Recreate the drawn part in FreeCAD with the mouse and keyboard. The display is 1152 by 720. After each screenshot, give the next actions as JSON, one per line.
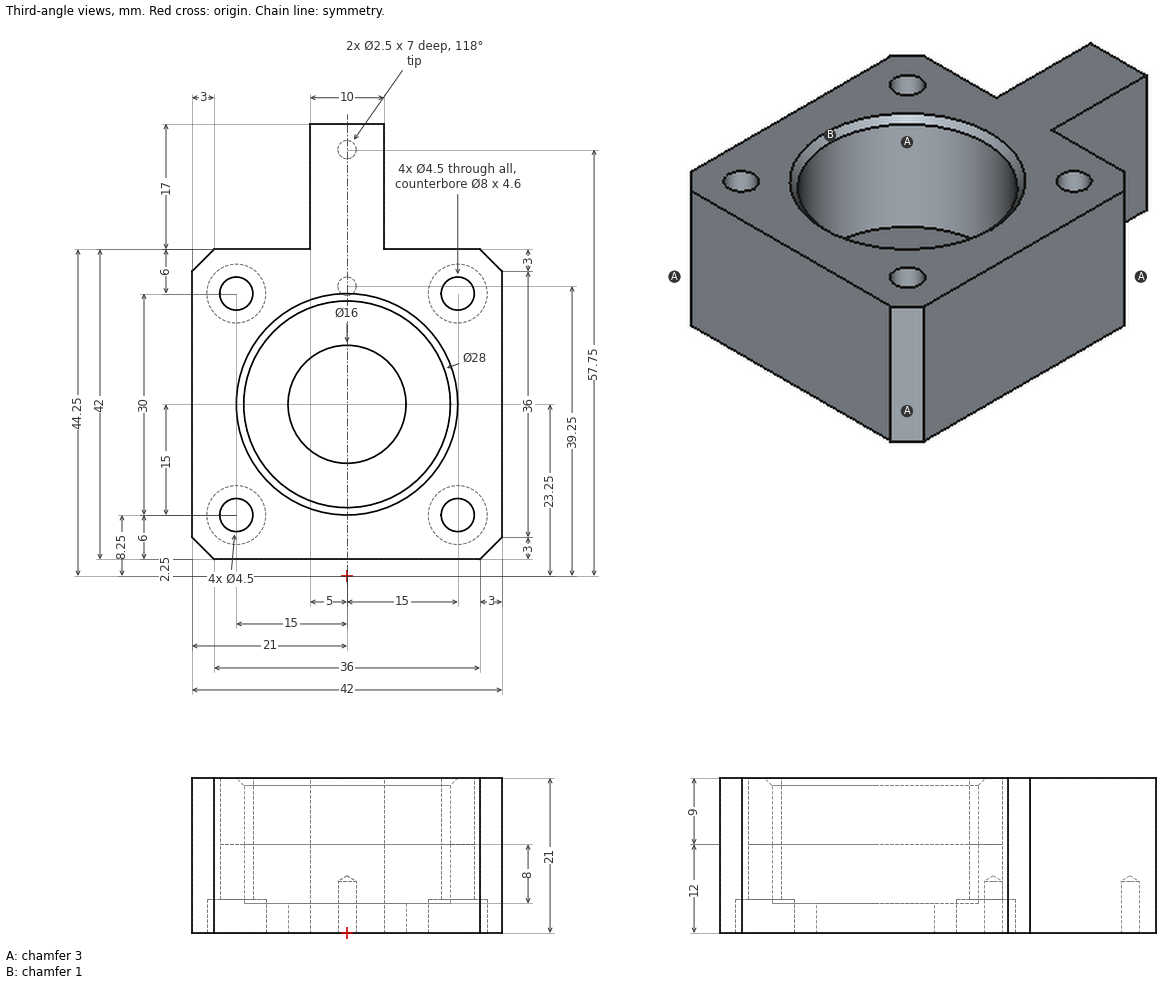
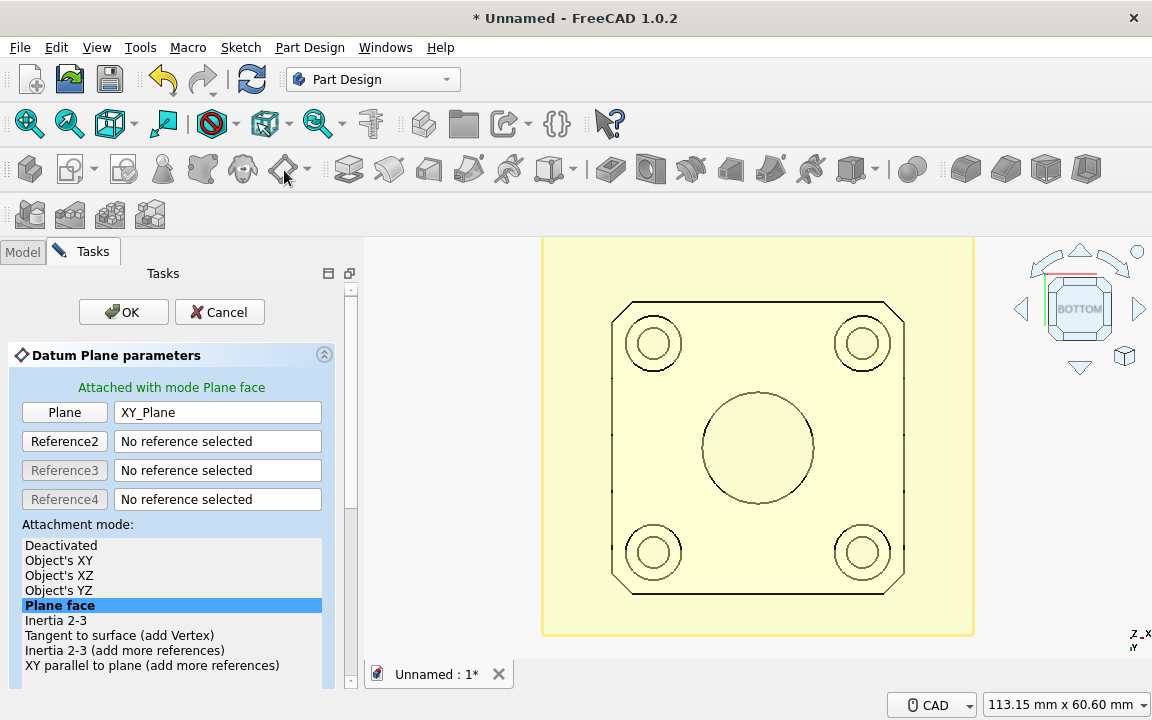
{"action": "scroll", "coordinate": [351, 486], "scroll_direction": "down", "scroll_amount": 4}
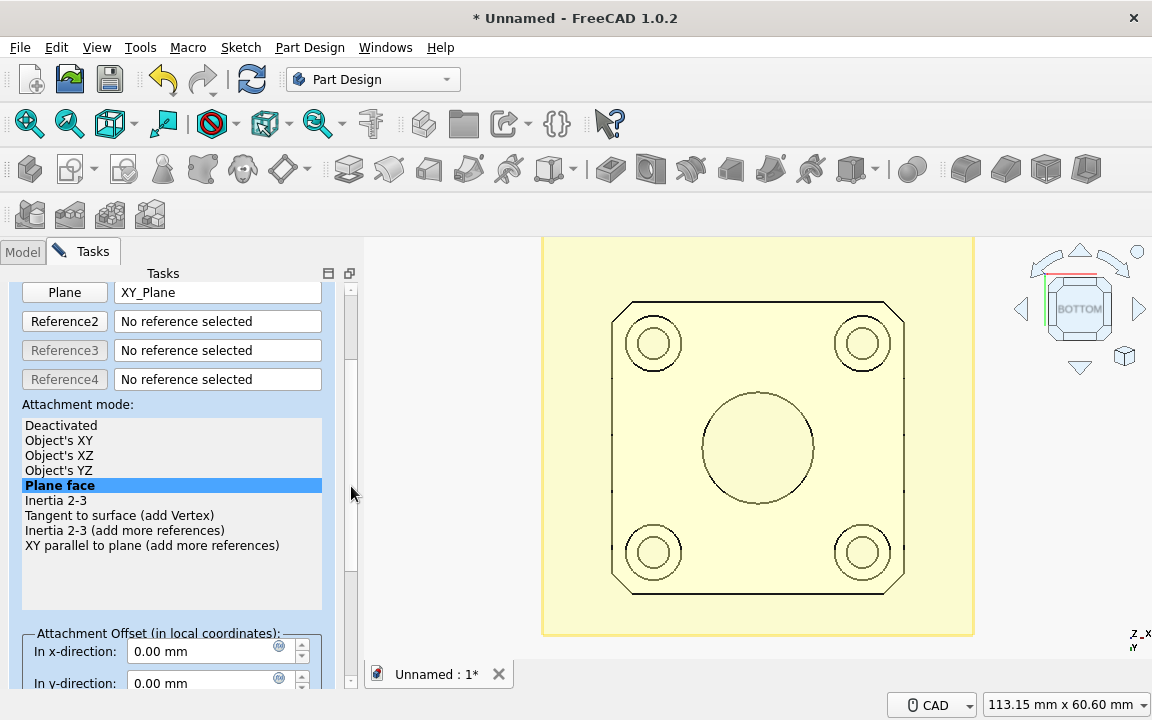
{"action": "triple_click", "coordinate": [210, 595]}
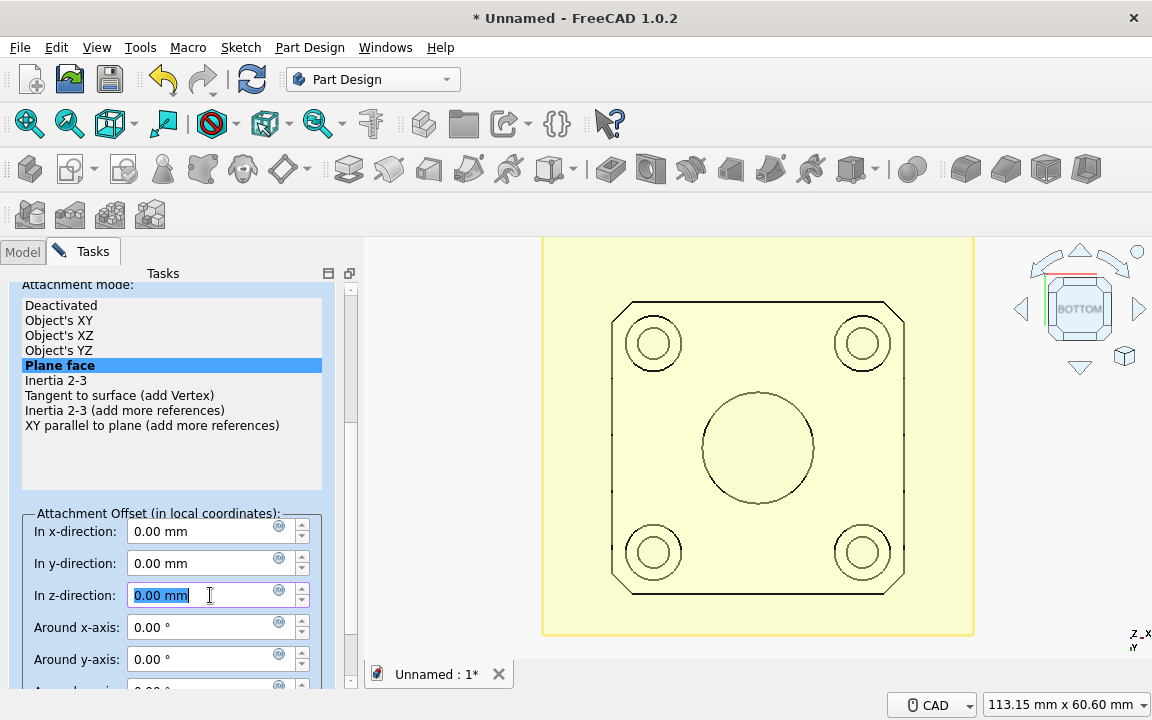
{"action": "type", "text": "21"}
{"action": "key", "text": "Tab"}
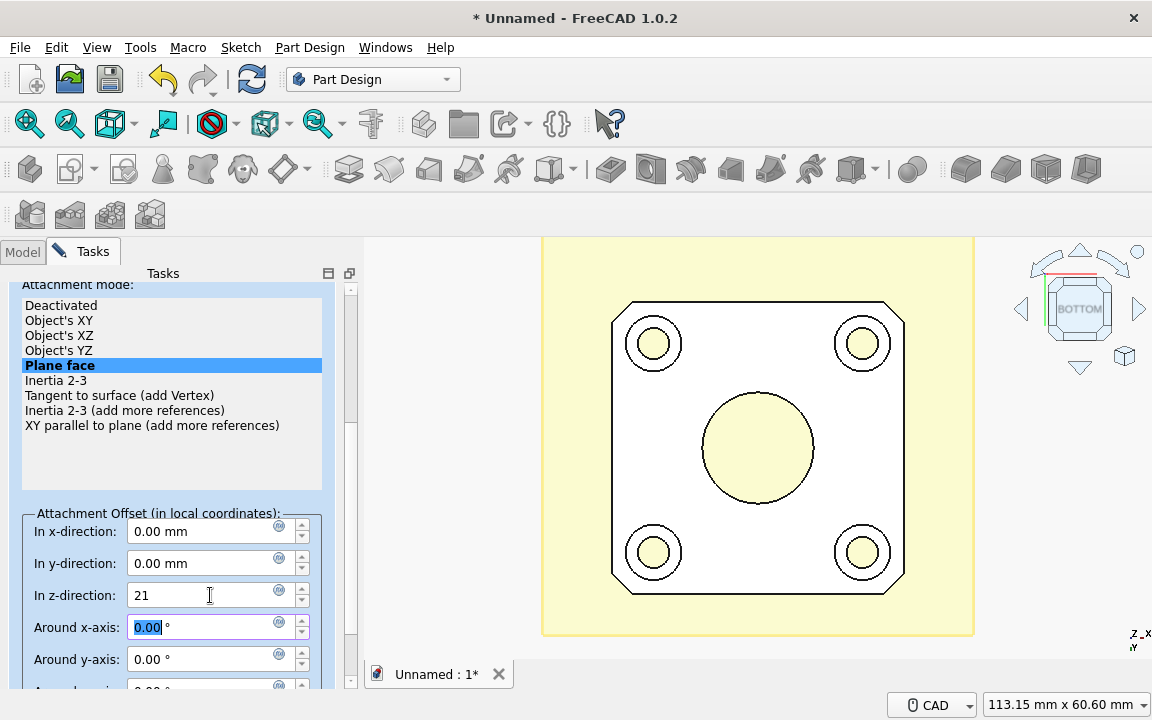
{"action": "scroll", "coordinate": [351, 486], "scroll_direction": "up", "scroll_amount": 5}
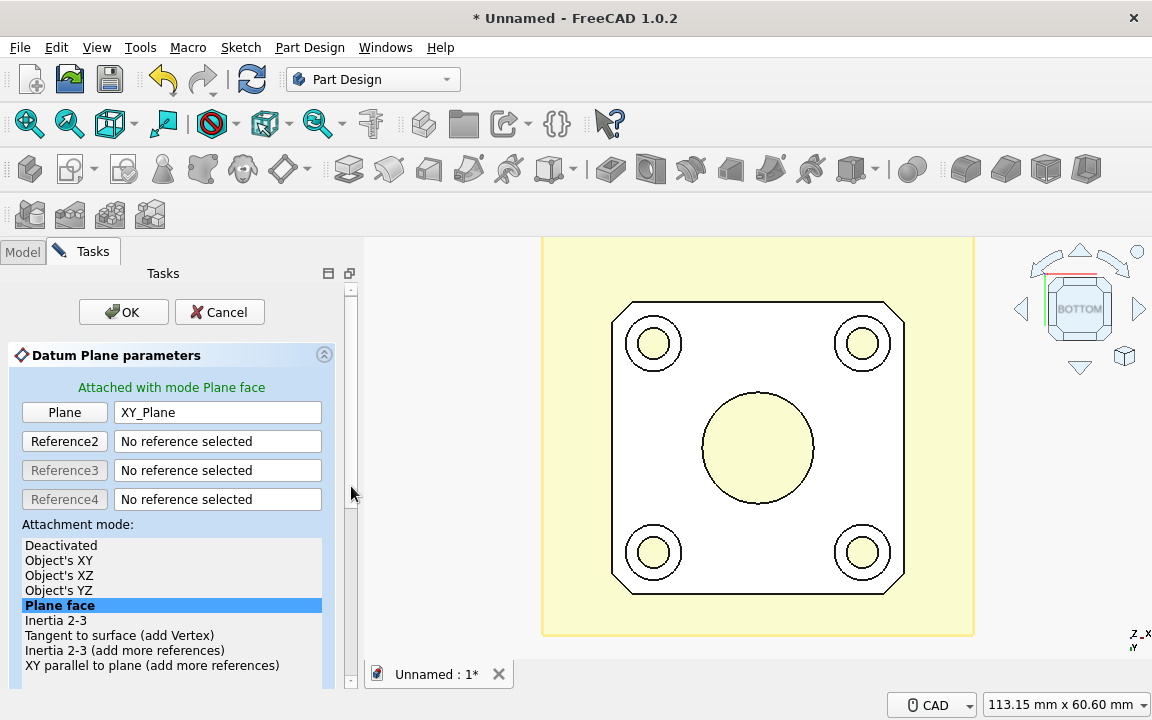
{"action": "left_click", "coordinate": [124, 312]}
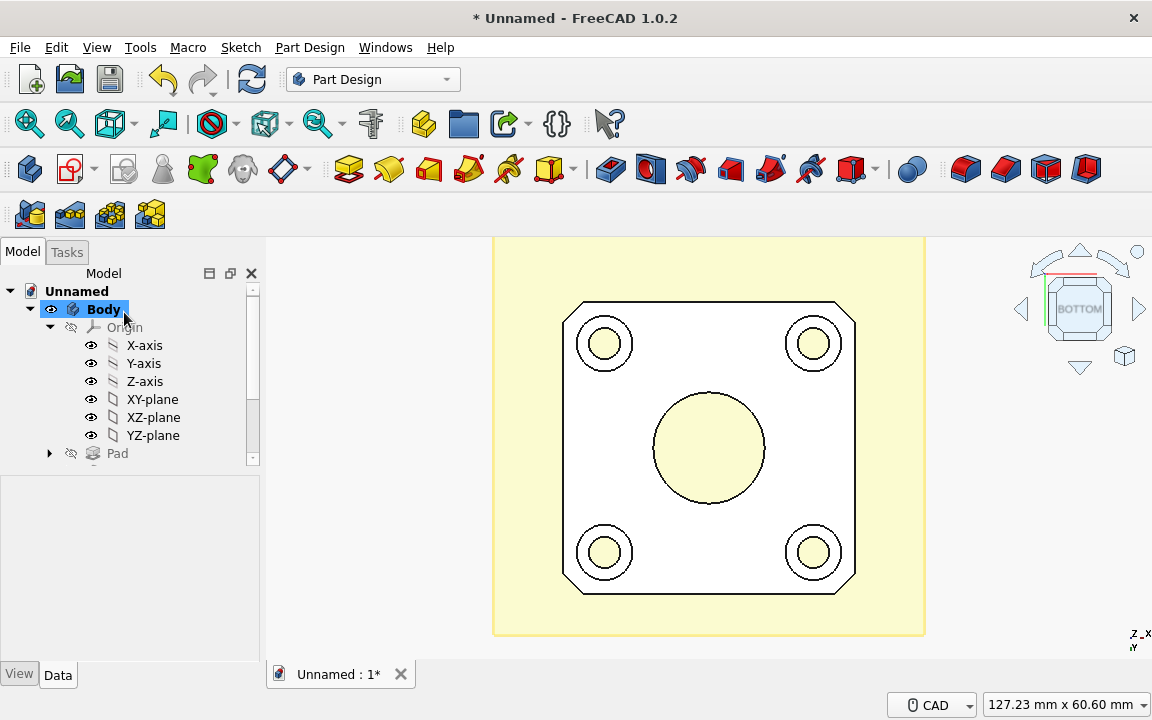
{"action": "scroll", "coordinate": [100, 377], "scroll_direction": "down", "scroll_amount": 3}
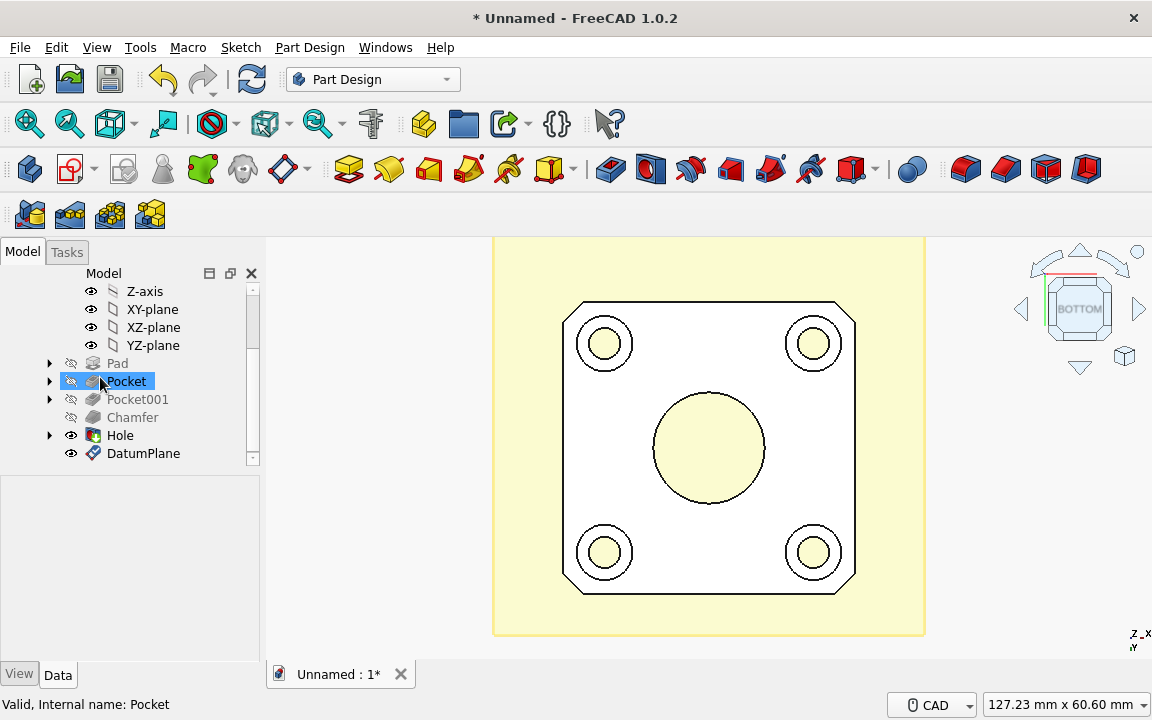
{"action": "left_click", "coordinate": [116, 453]}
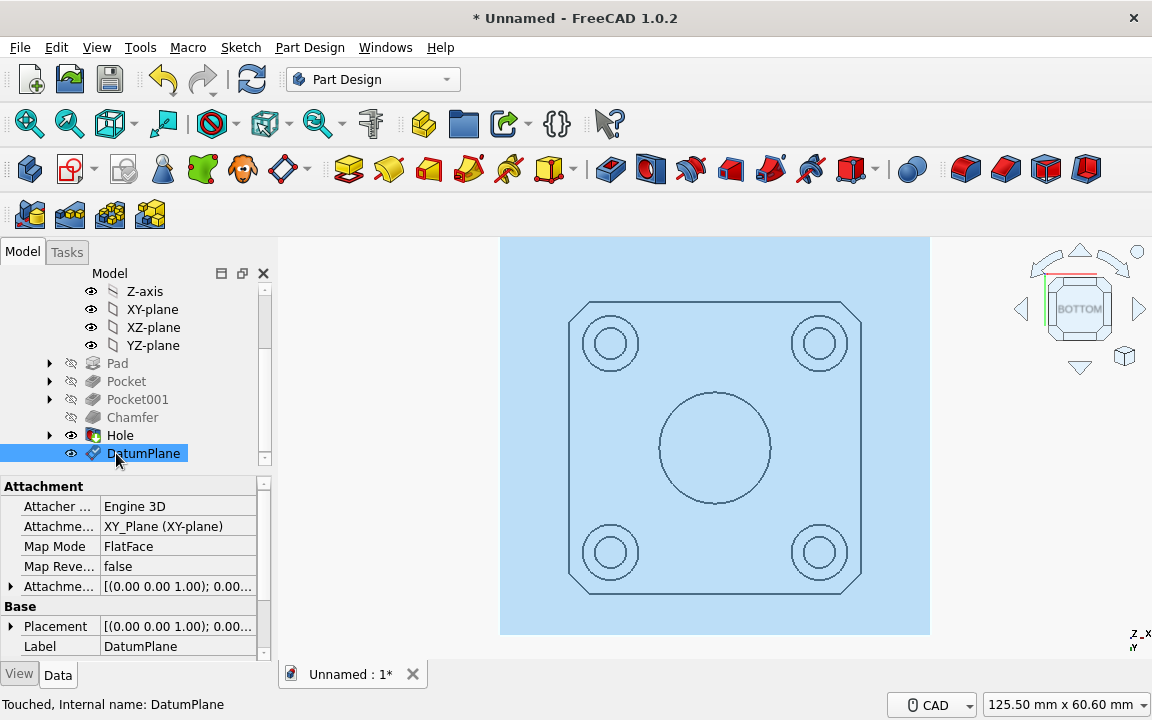
{"action": "left_click", "coordinate": [70, 170]}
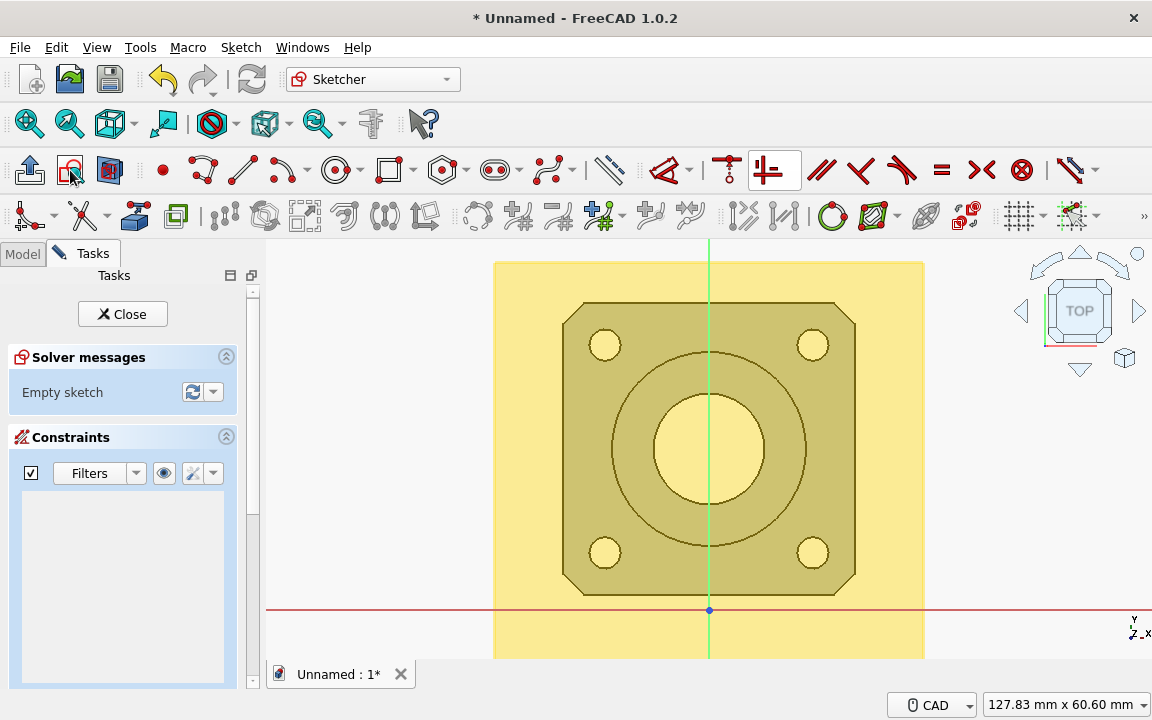
{"action": "scroll", "coordinate": [331, 414], "scroll_direction": "down", "scroll_amount": 1}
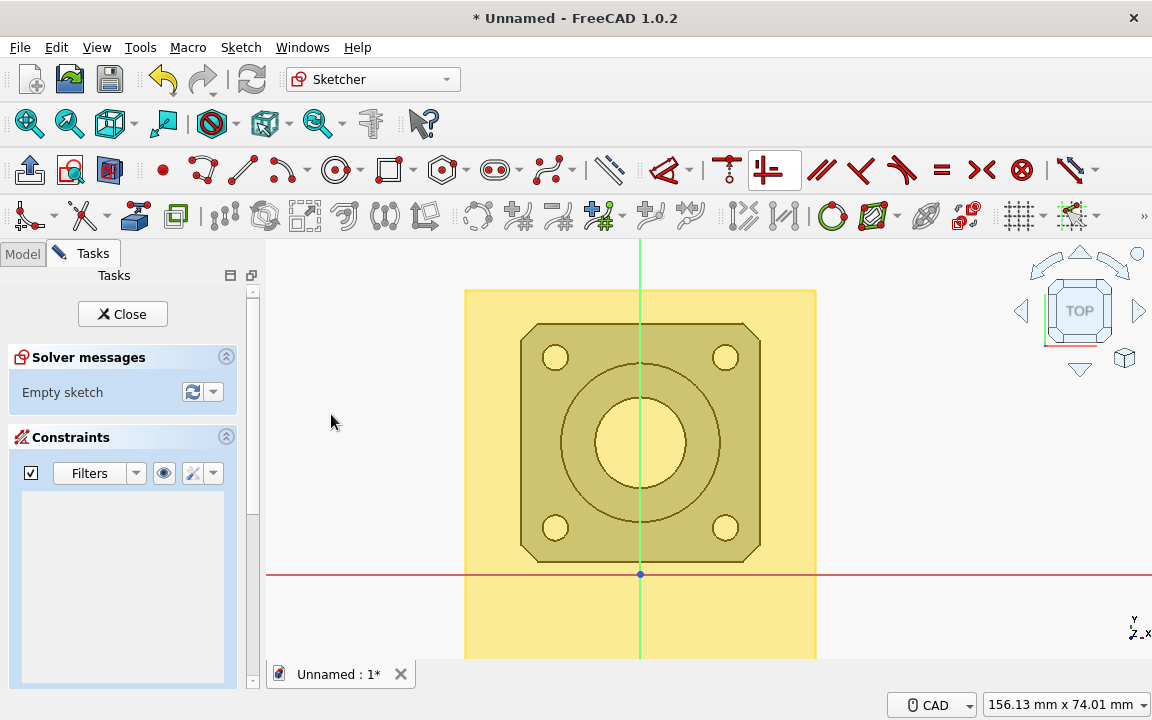
{"action": "left_click", "coordinate": [204, 170]}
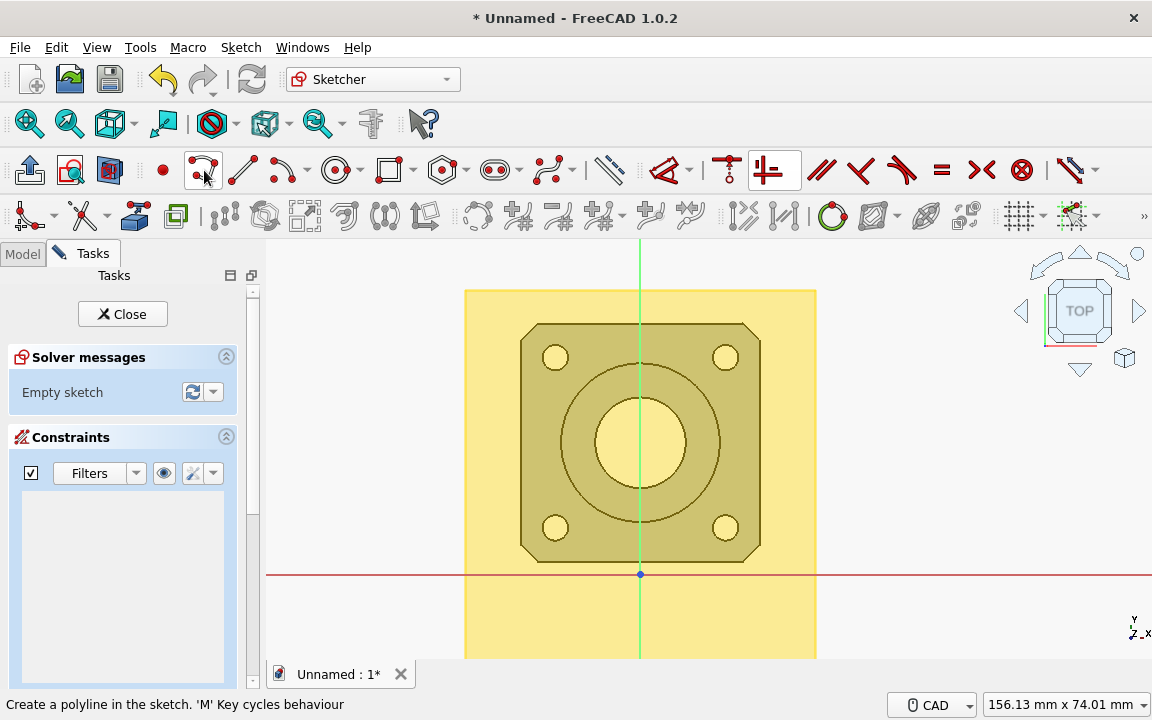
{"action": "scroll", "coordinate": [538, 562], "scroll_direction": "up", "scroll_amount": 2}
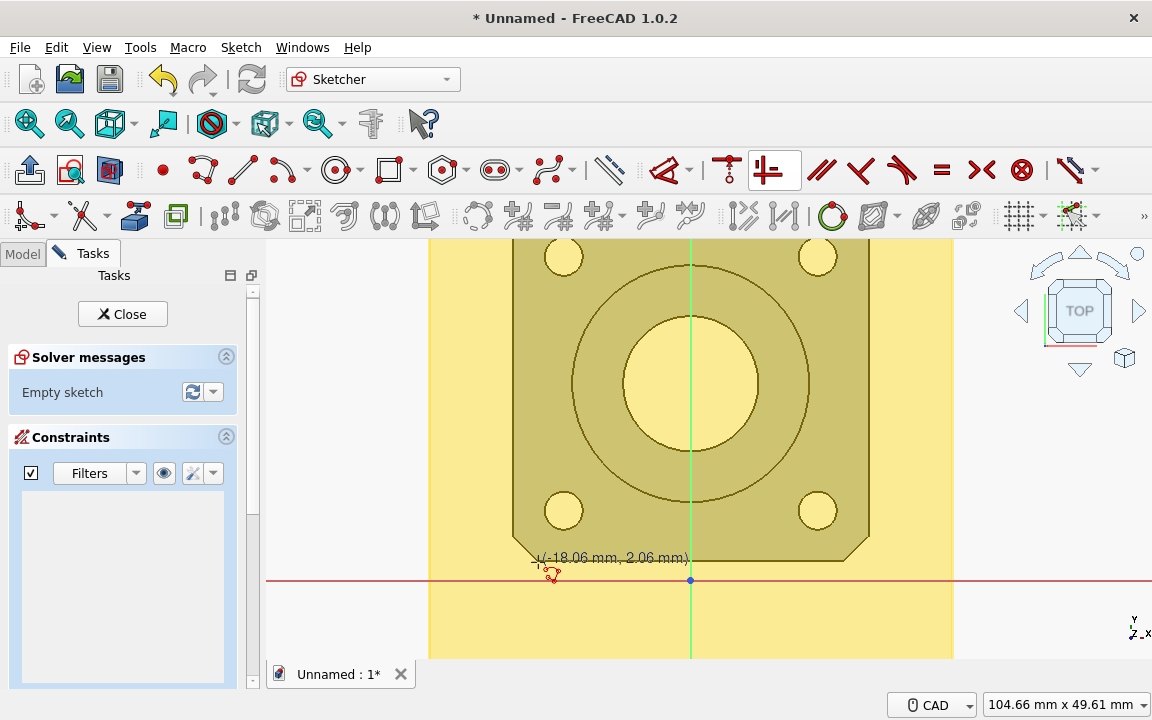
{"action": "left_click", "coordinate": [538, 561]}
{"action": "left_click", "coordinate": [843, 561]}
{"action": "left_click", "coordinate": [869, 536]}